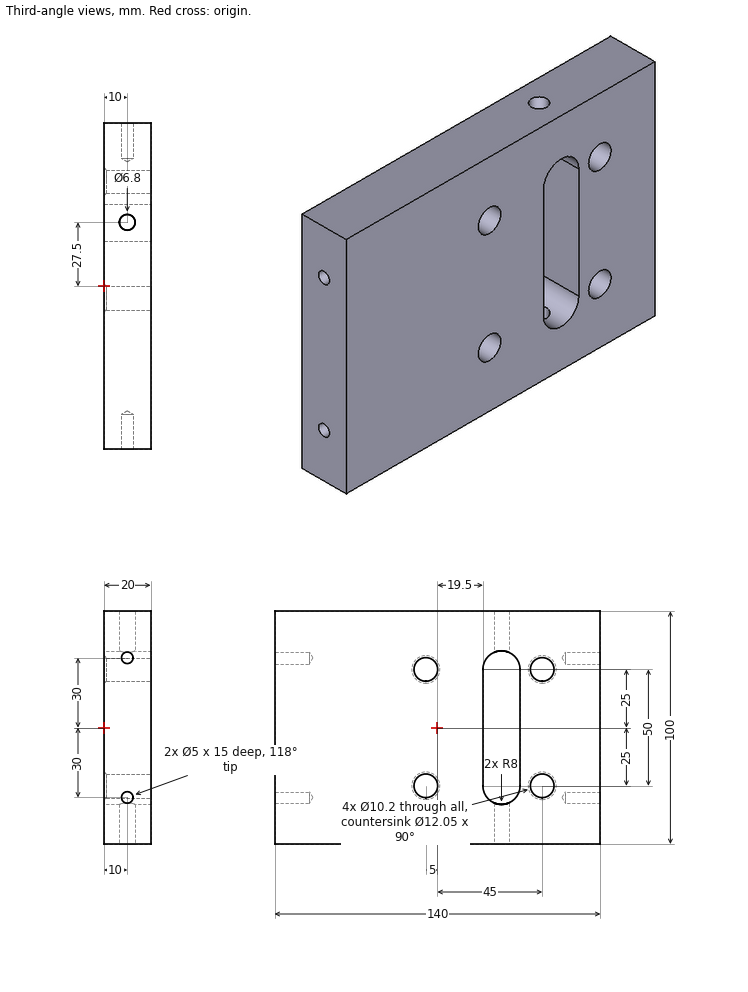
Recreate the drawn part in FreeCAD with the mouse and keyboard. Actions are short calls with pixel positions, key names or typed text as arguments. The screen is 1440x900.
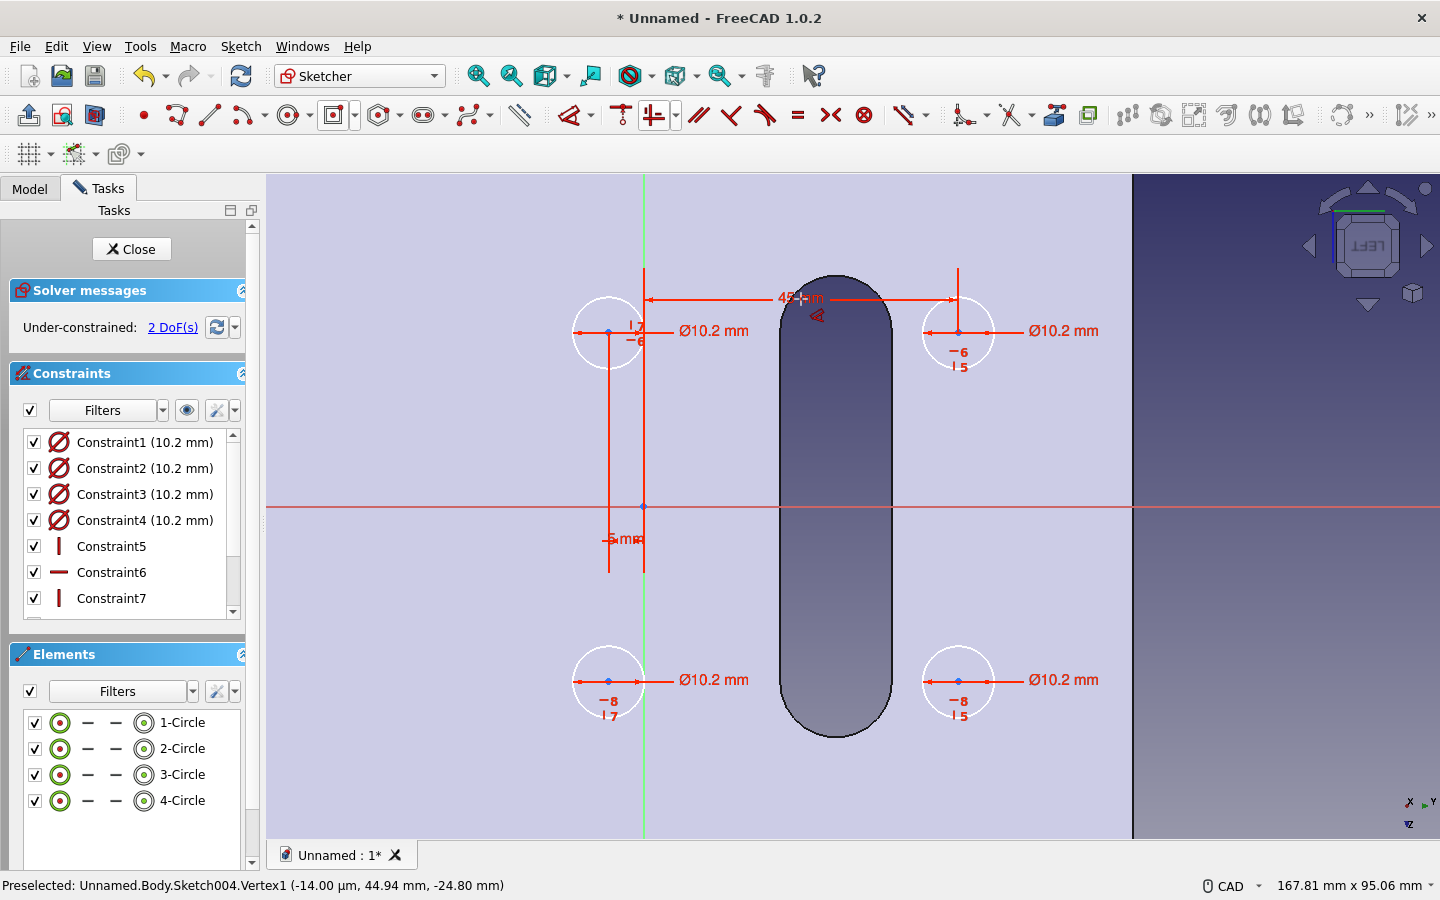
click(958, 333)
click(992, 420)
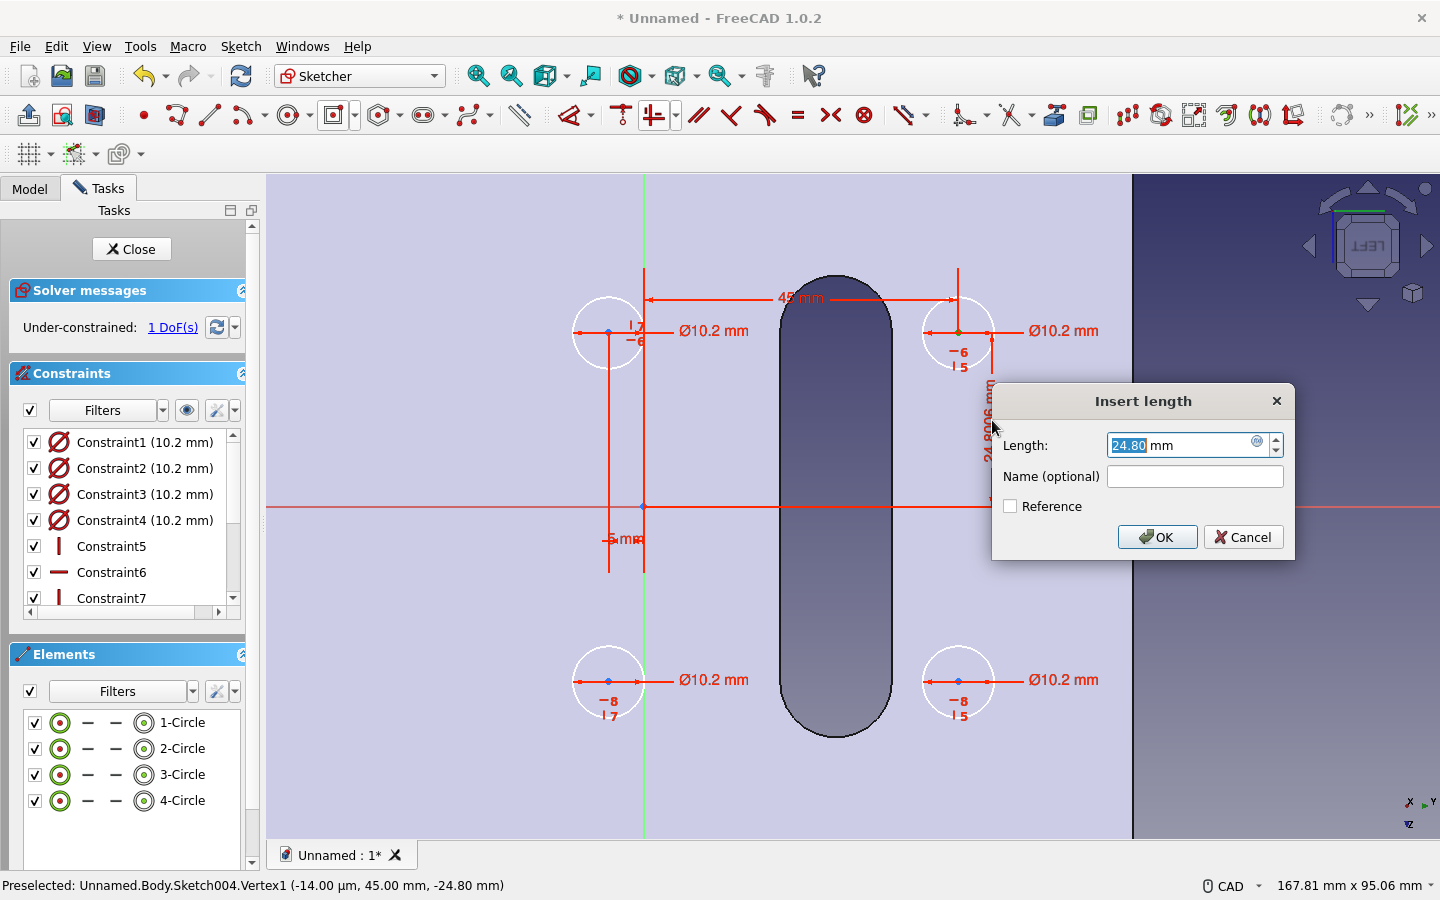
text(25)
key(Return)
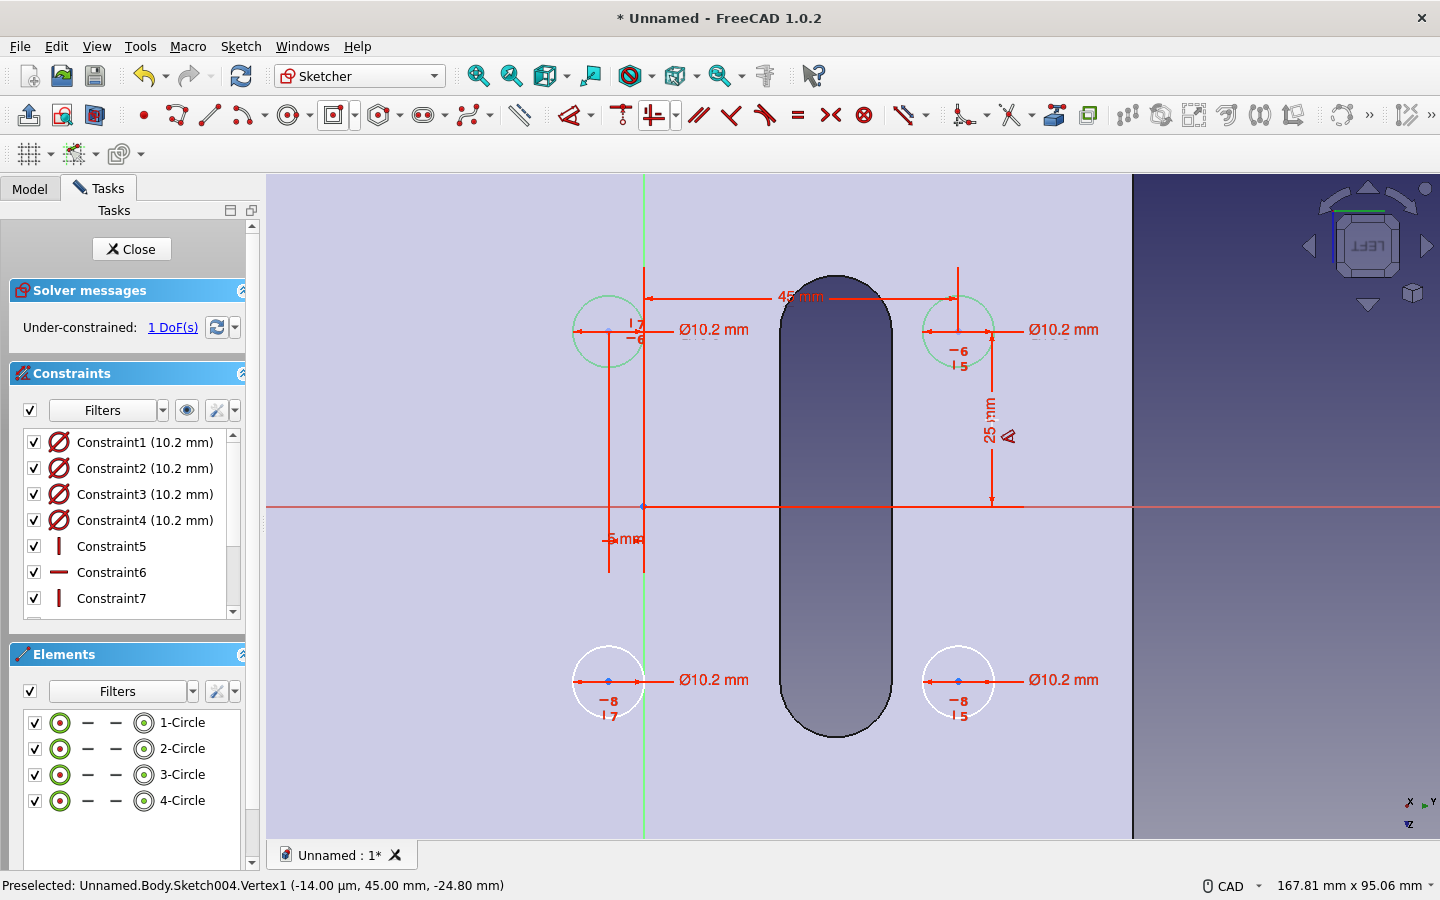
click(958, 682)
click(992, 594)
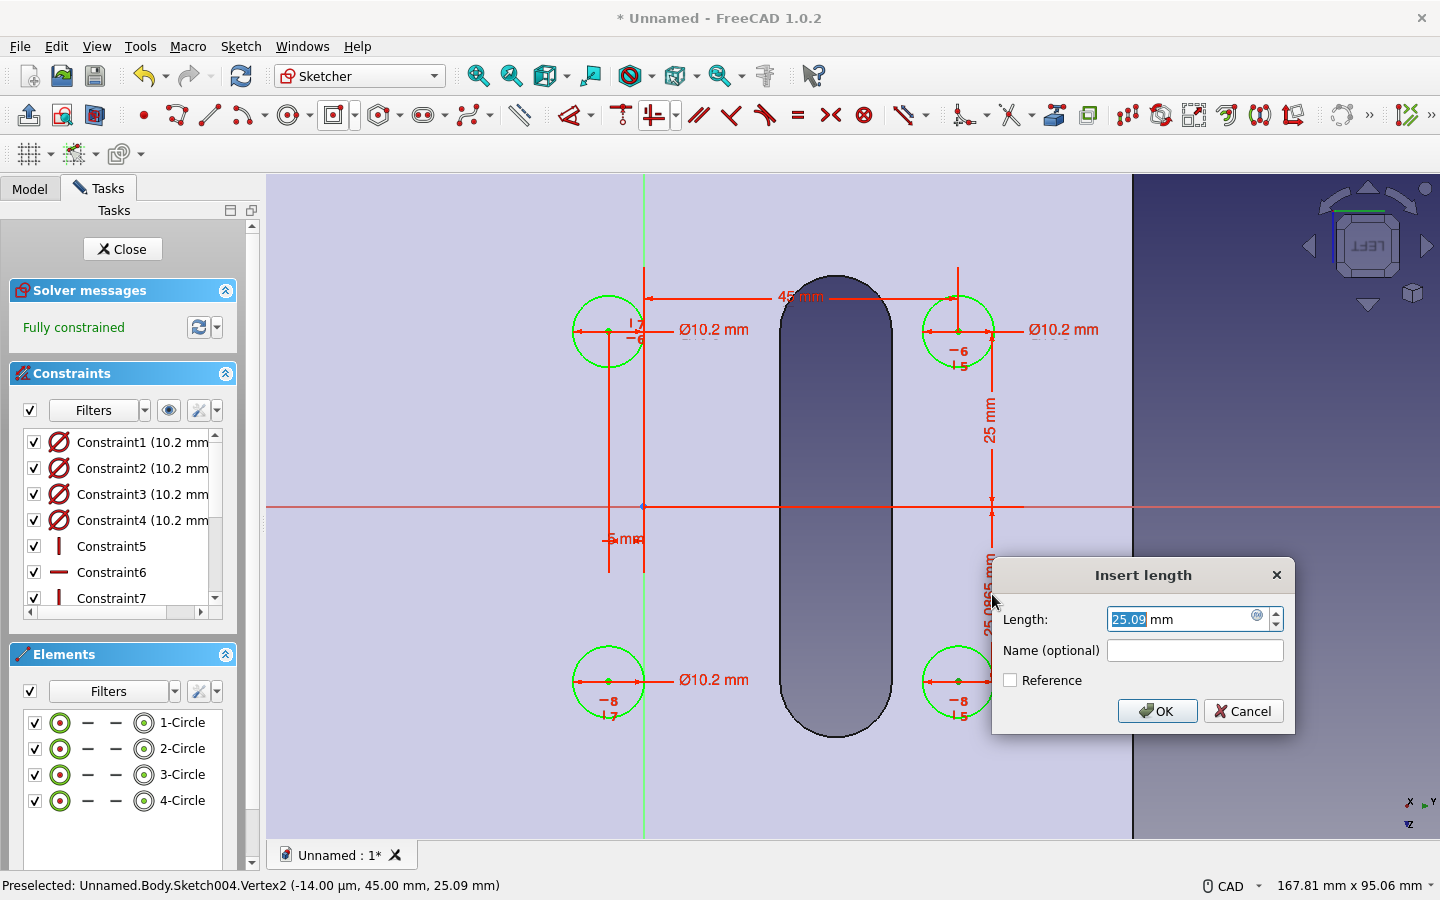
text(25)
key(Return)
key(Escape)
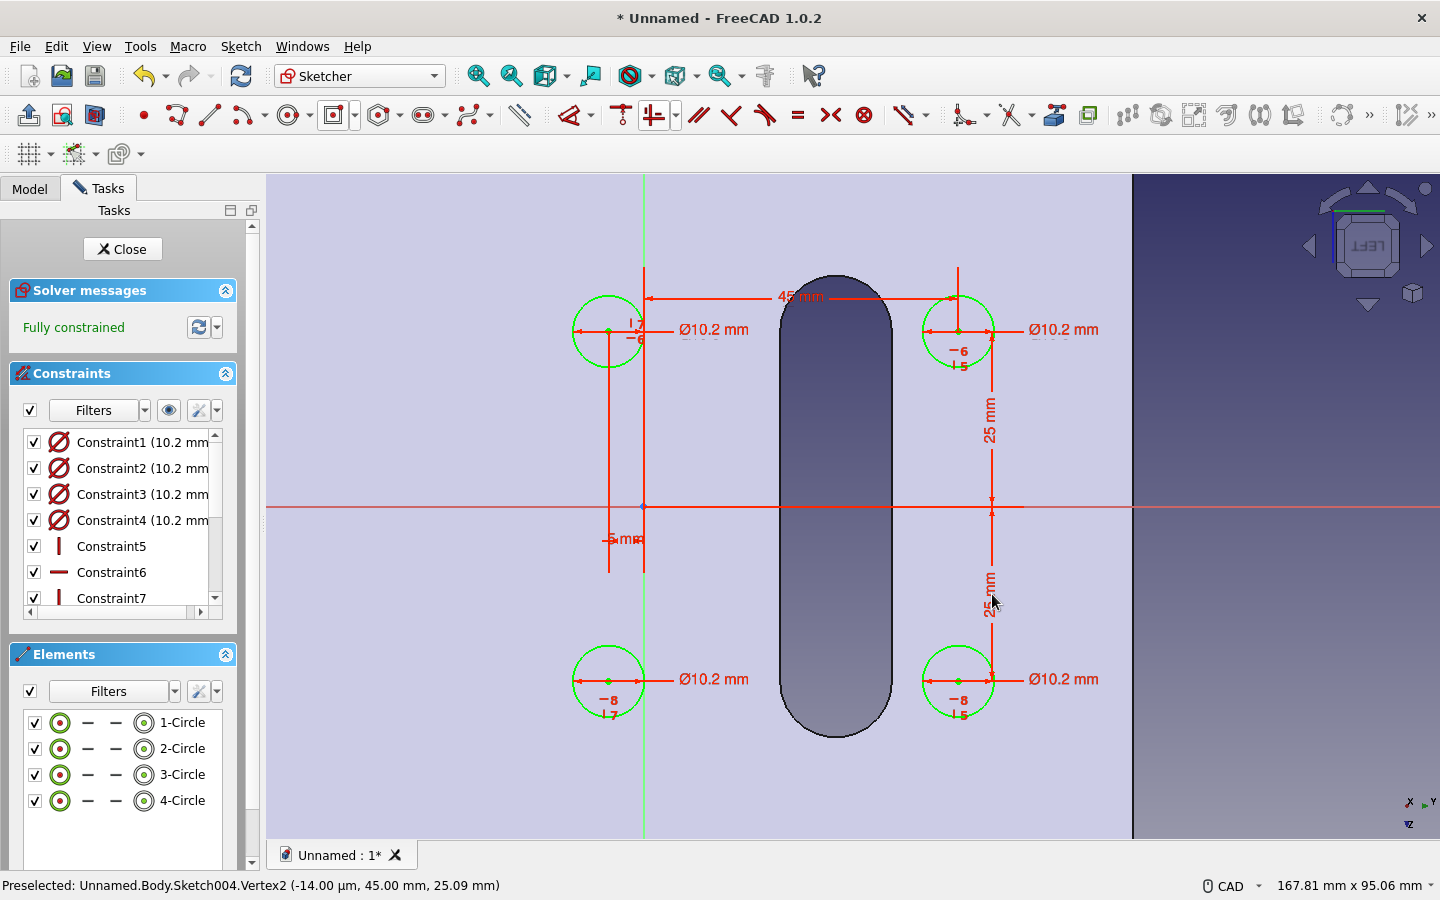
click(123, 249)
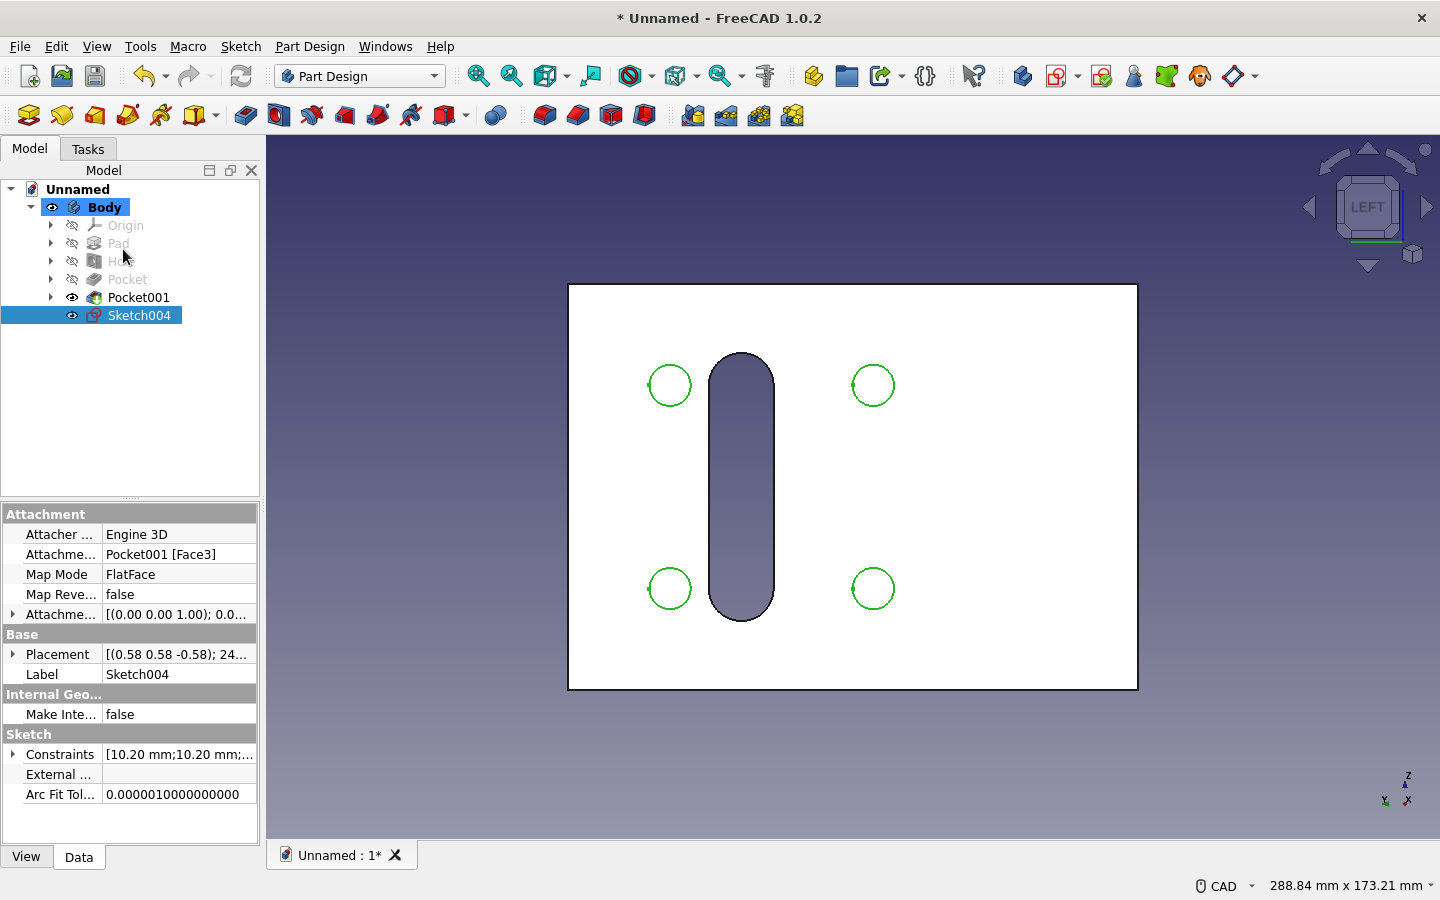
click(279, 116)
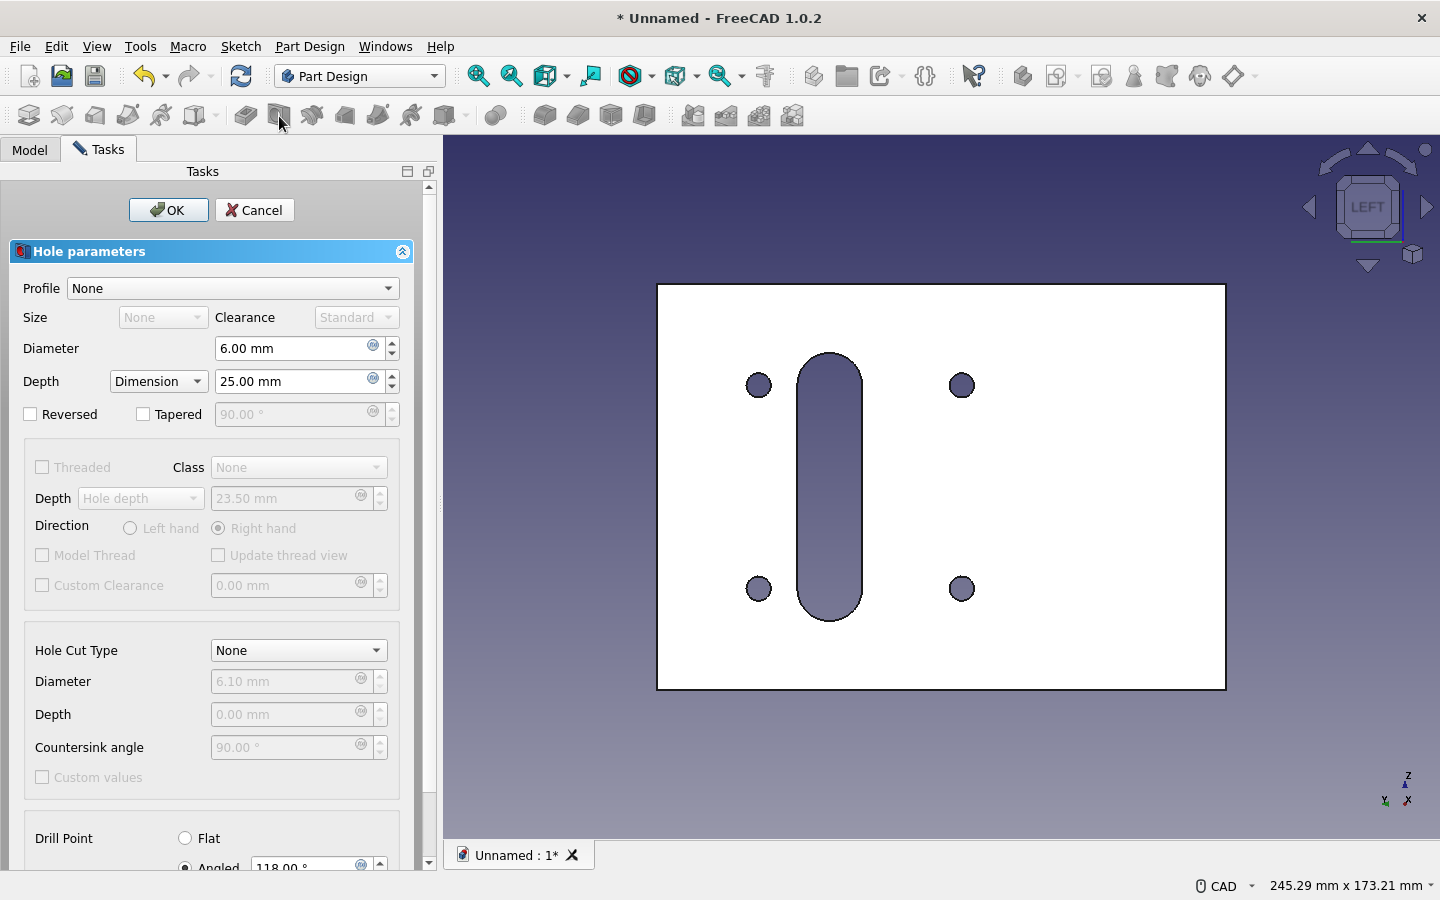
triple_click(300, 348)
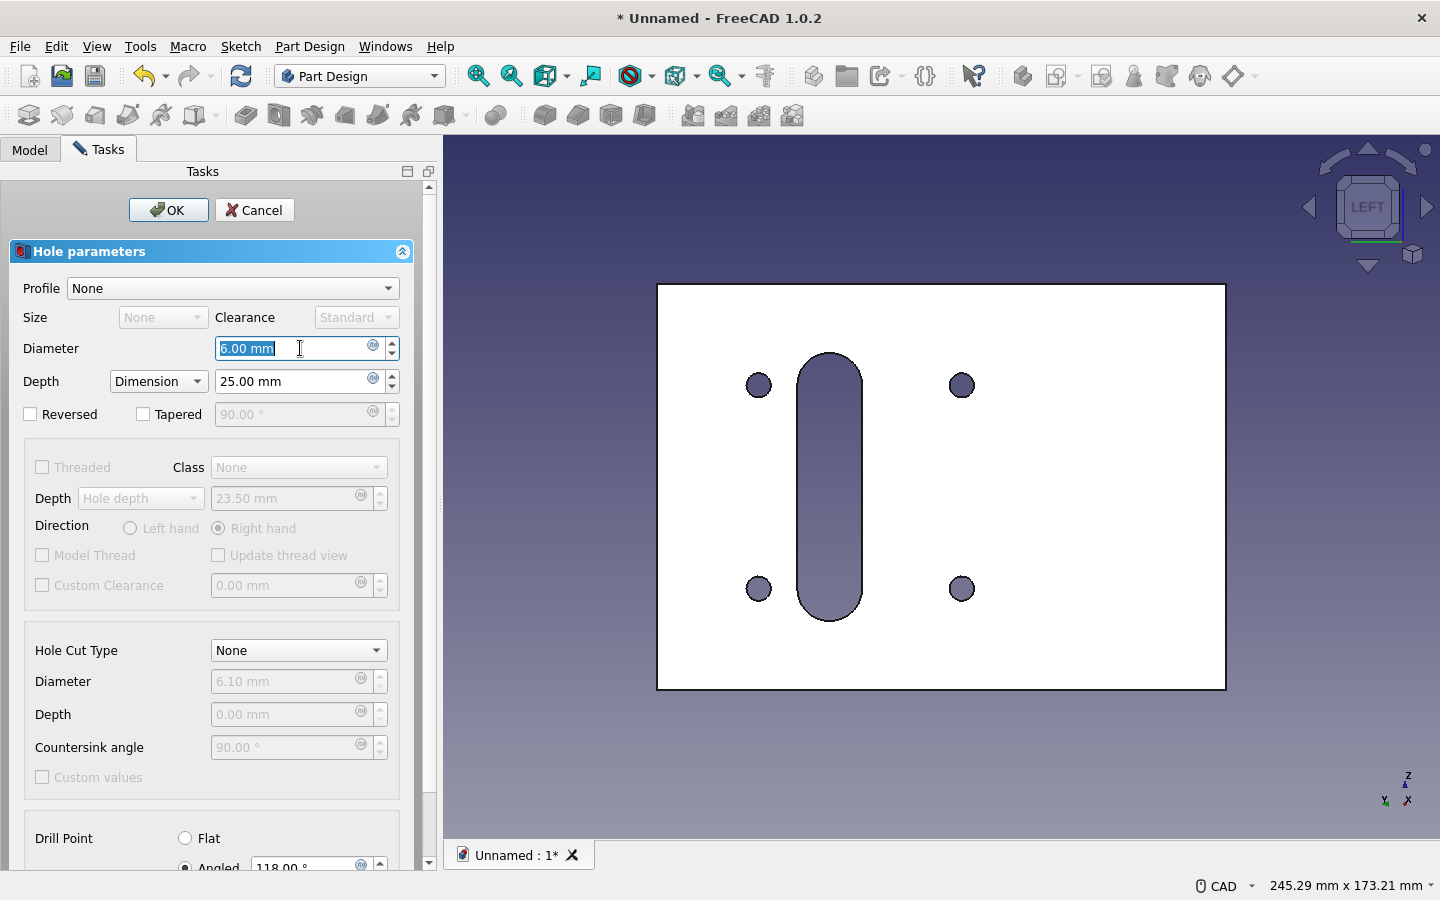
text(10.2)
key(Tab)